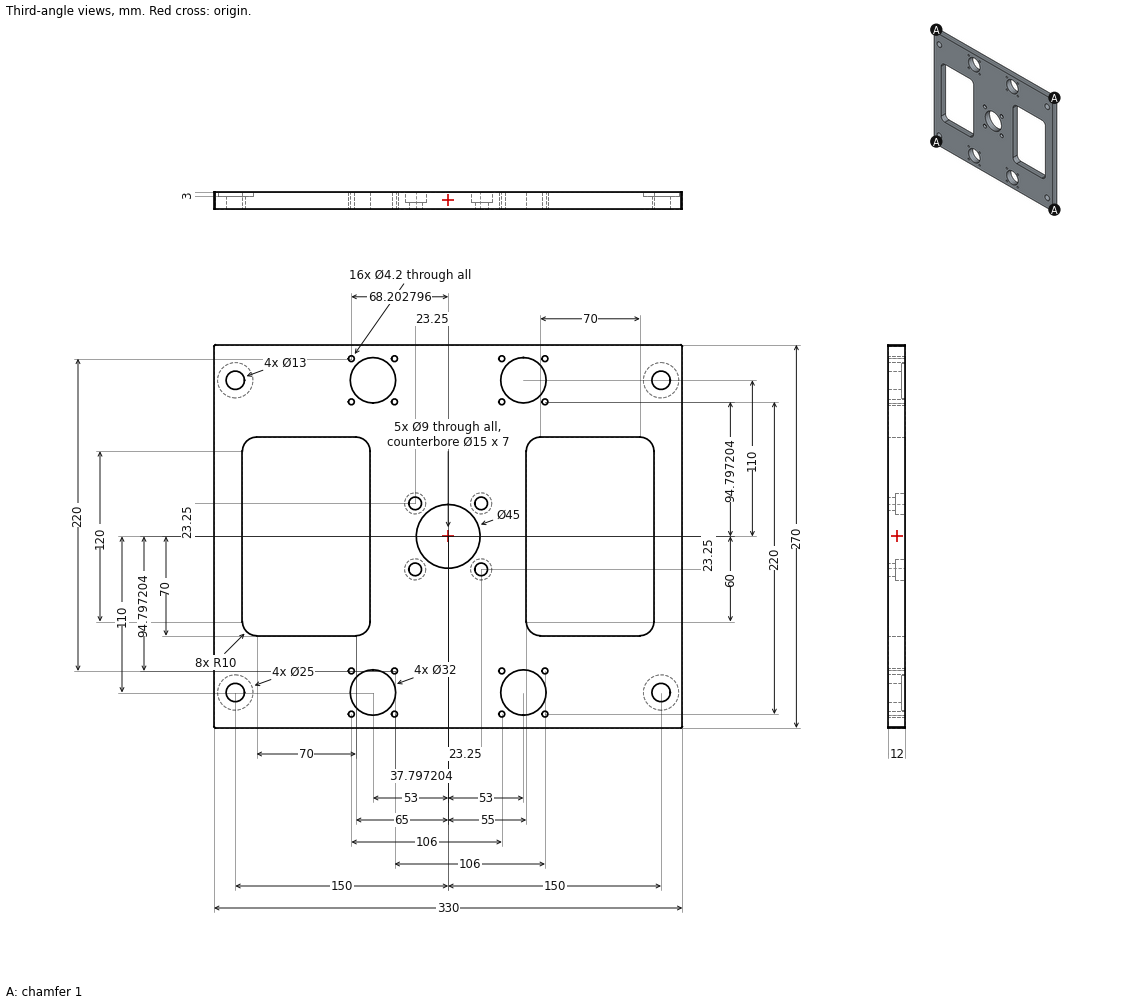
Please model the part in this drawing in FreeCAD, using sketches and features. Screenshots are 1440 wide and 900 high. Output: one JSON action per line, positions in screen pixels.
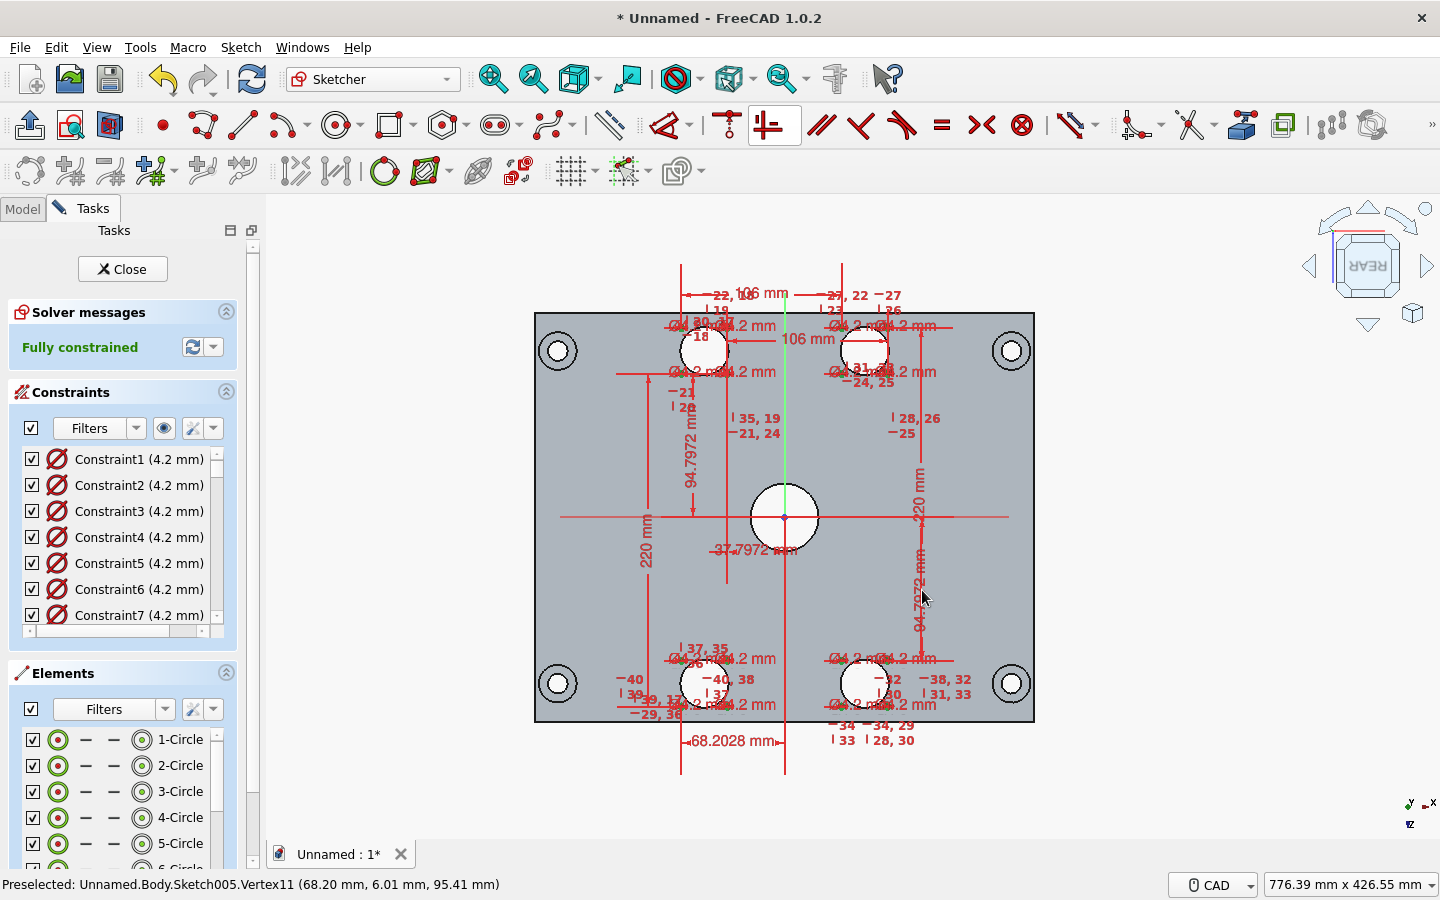
{"action": "left_click", "coordinate": [123, 269]}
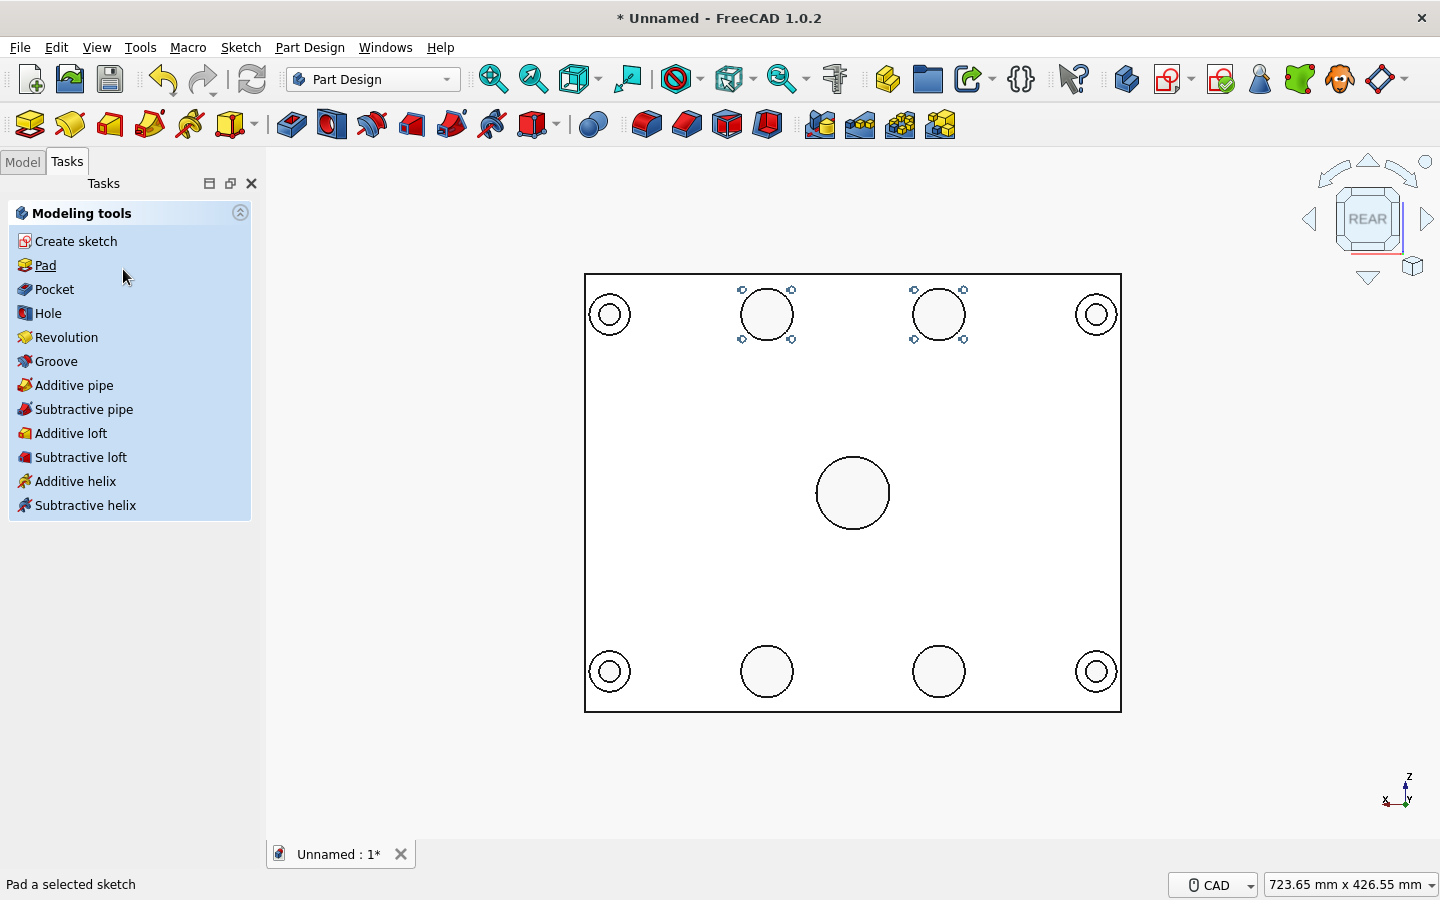
{"action": "left_click", "coordinate": [332, 124]}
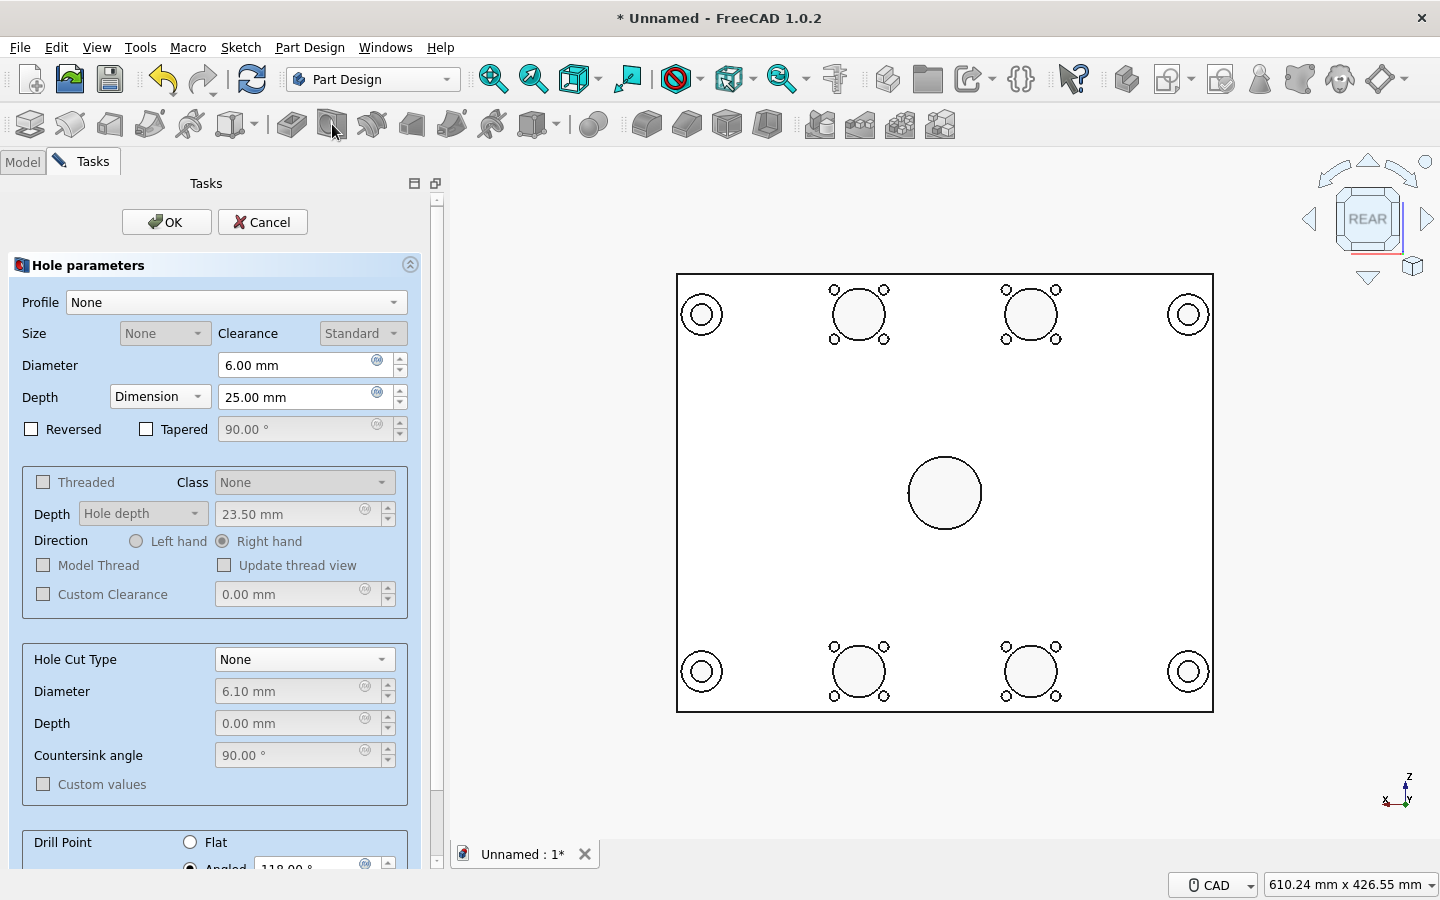
{"action": "triple_click", "coordinate": [305, 365]}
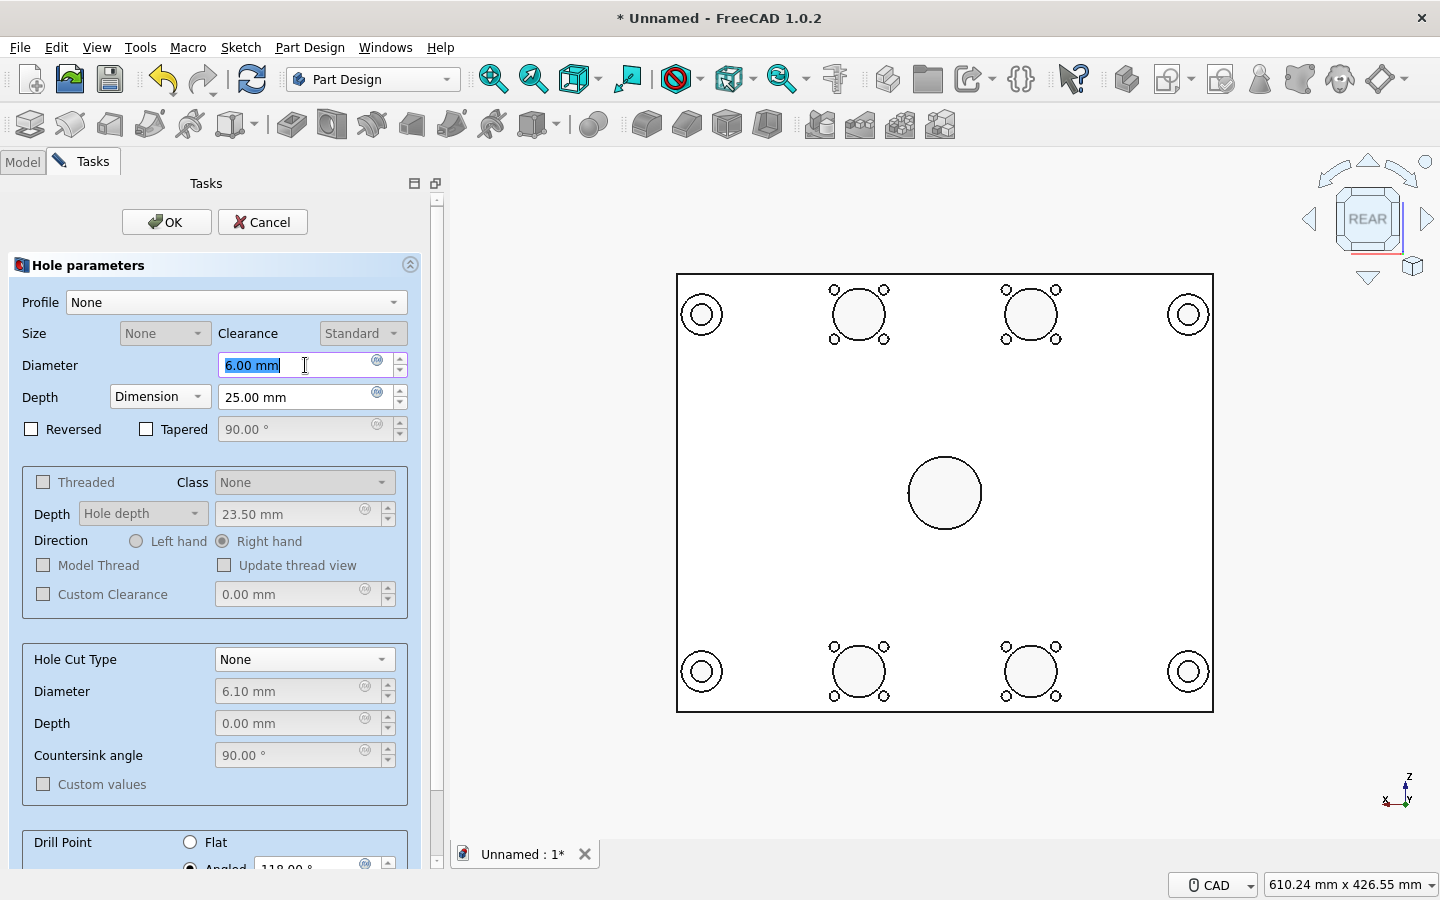
{"action": "type", "text": "4.2"}
{"action": "key", "text": "Tab"}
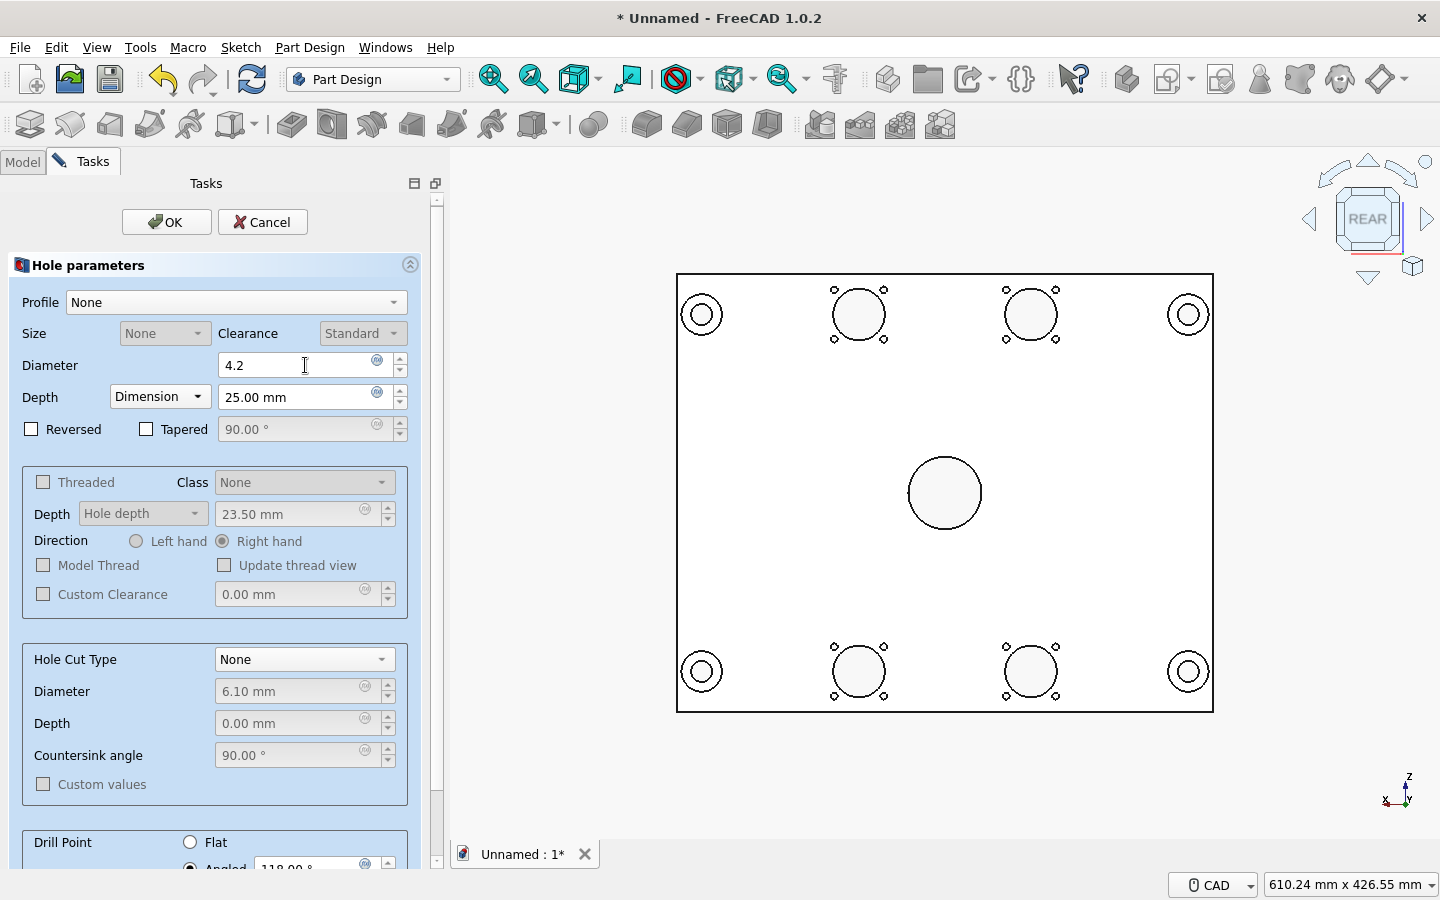
{"action": "left_click", "coordinate": [161, 396]}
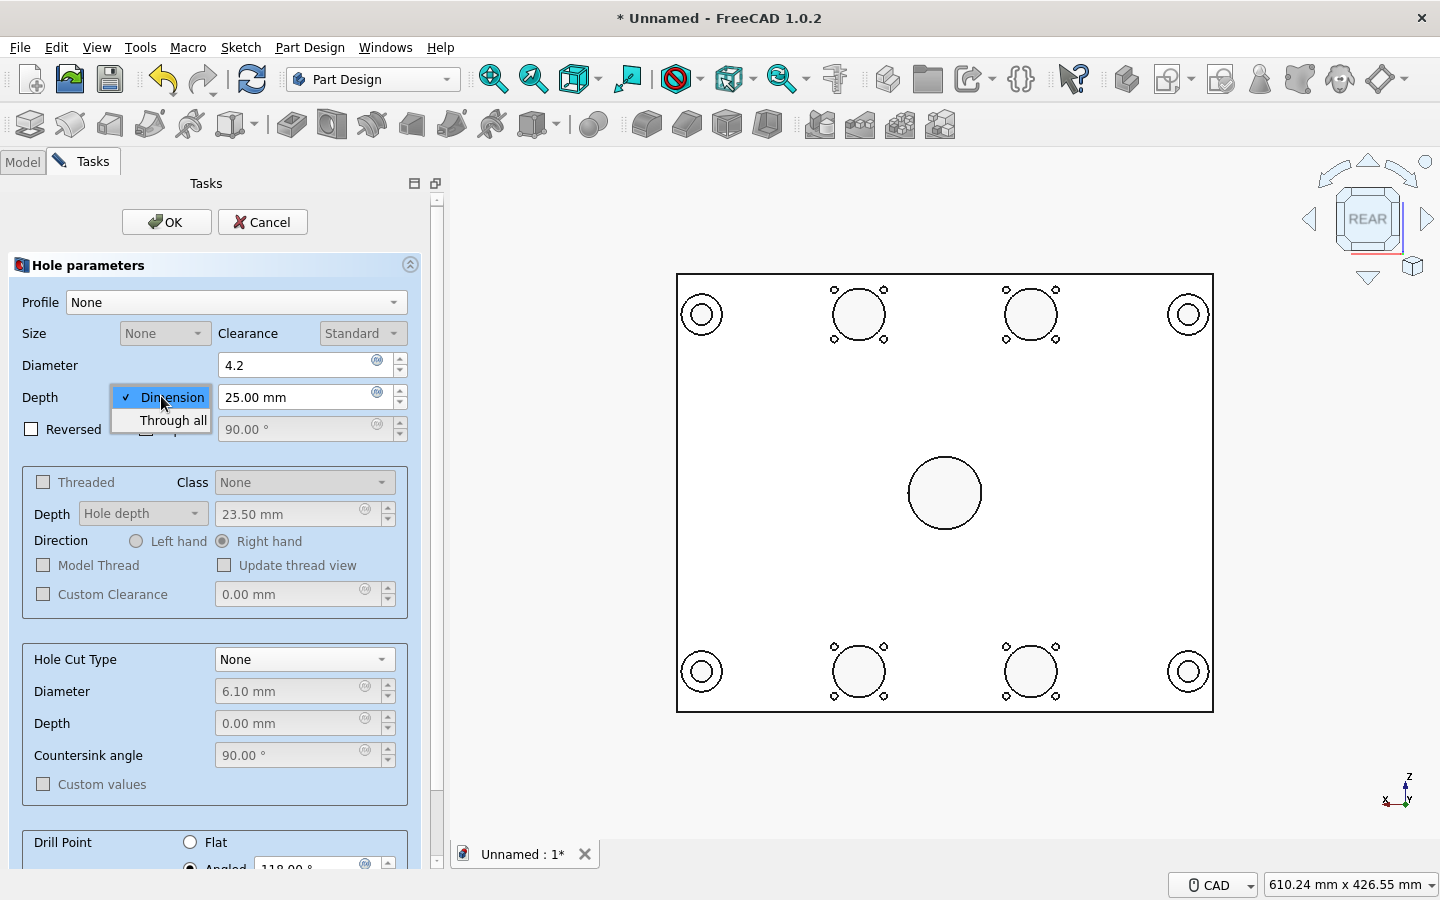
{"action": "left_click", "coordinate": [160, 420]}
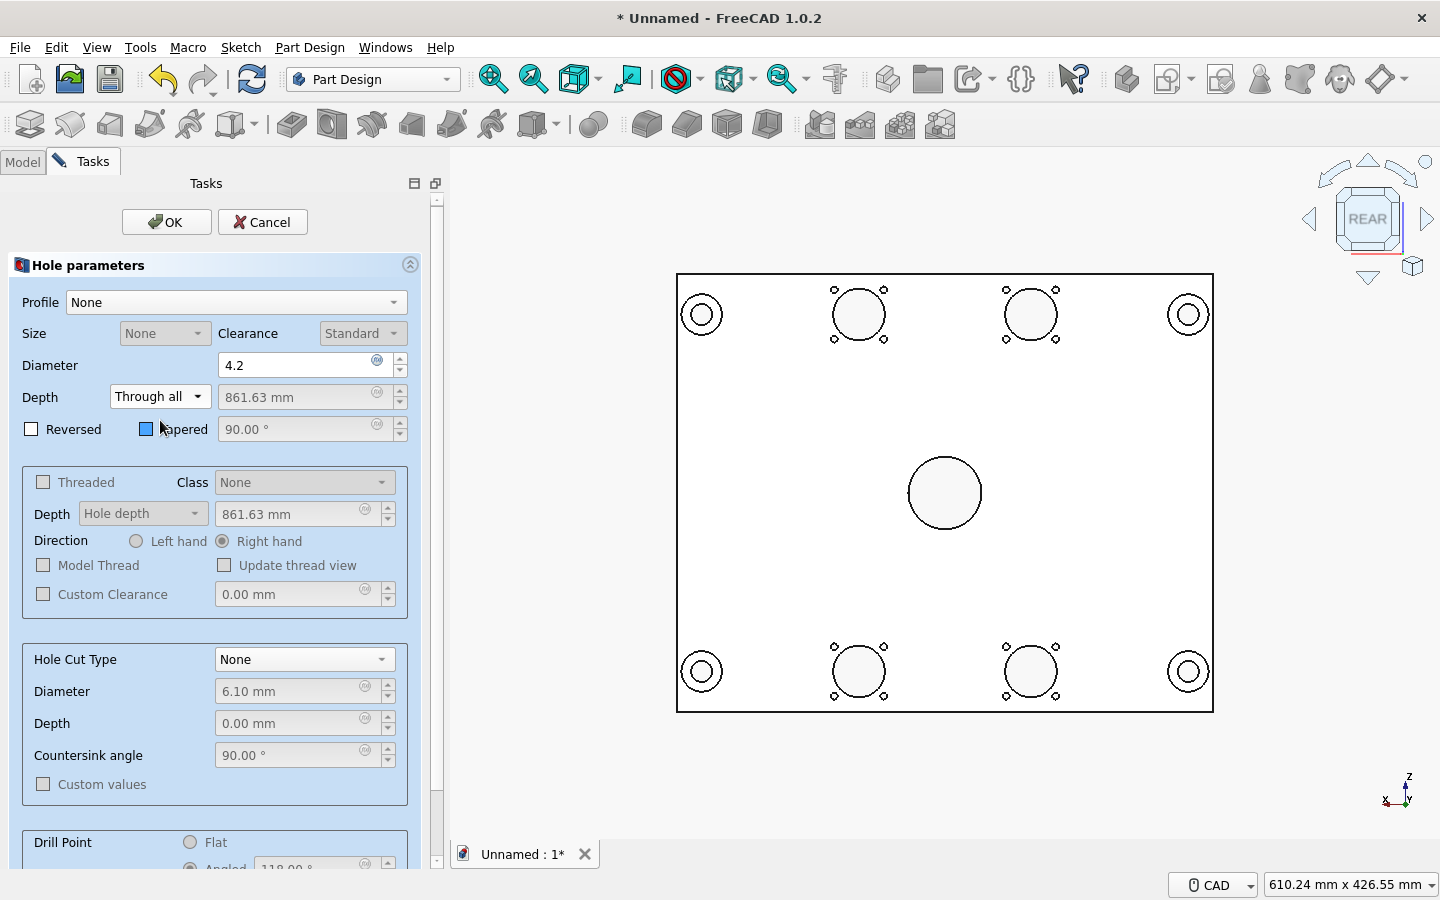
{"action": "left_click", "coordinate": [167, 222]}